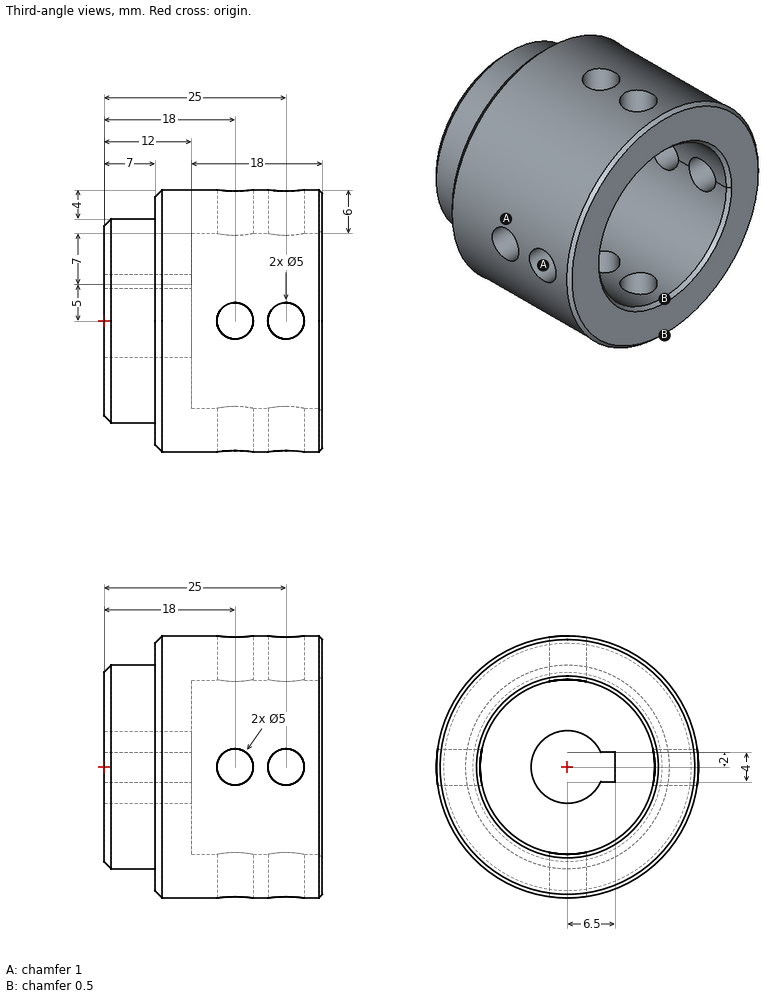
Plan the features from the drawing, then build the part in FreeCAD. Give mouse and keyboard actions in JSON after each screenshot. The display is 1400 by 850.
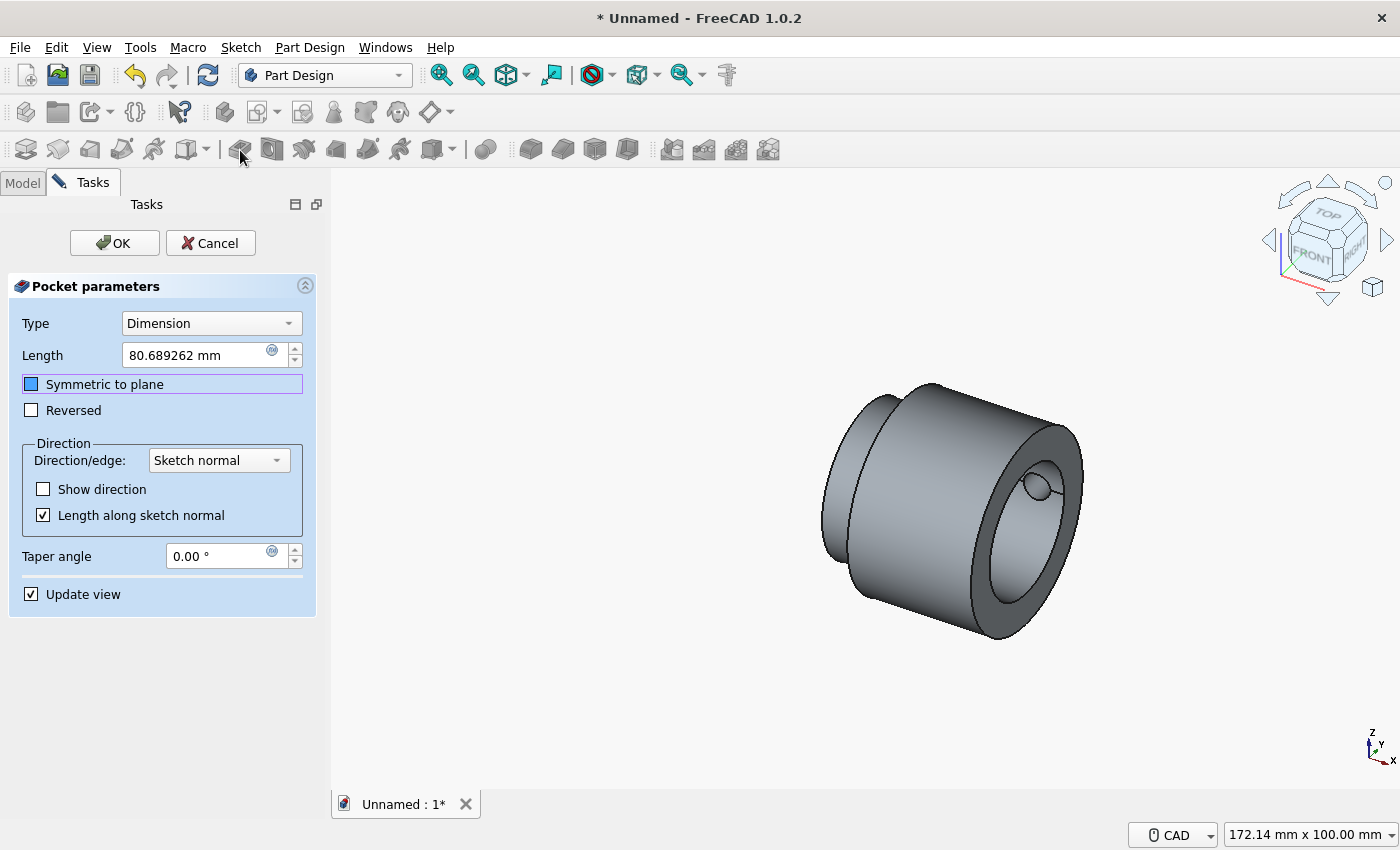
{"action": "left_click", "coordinate": [30, 384]}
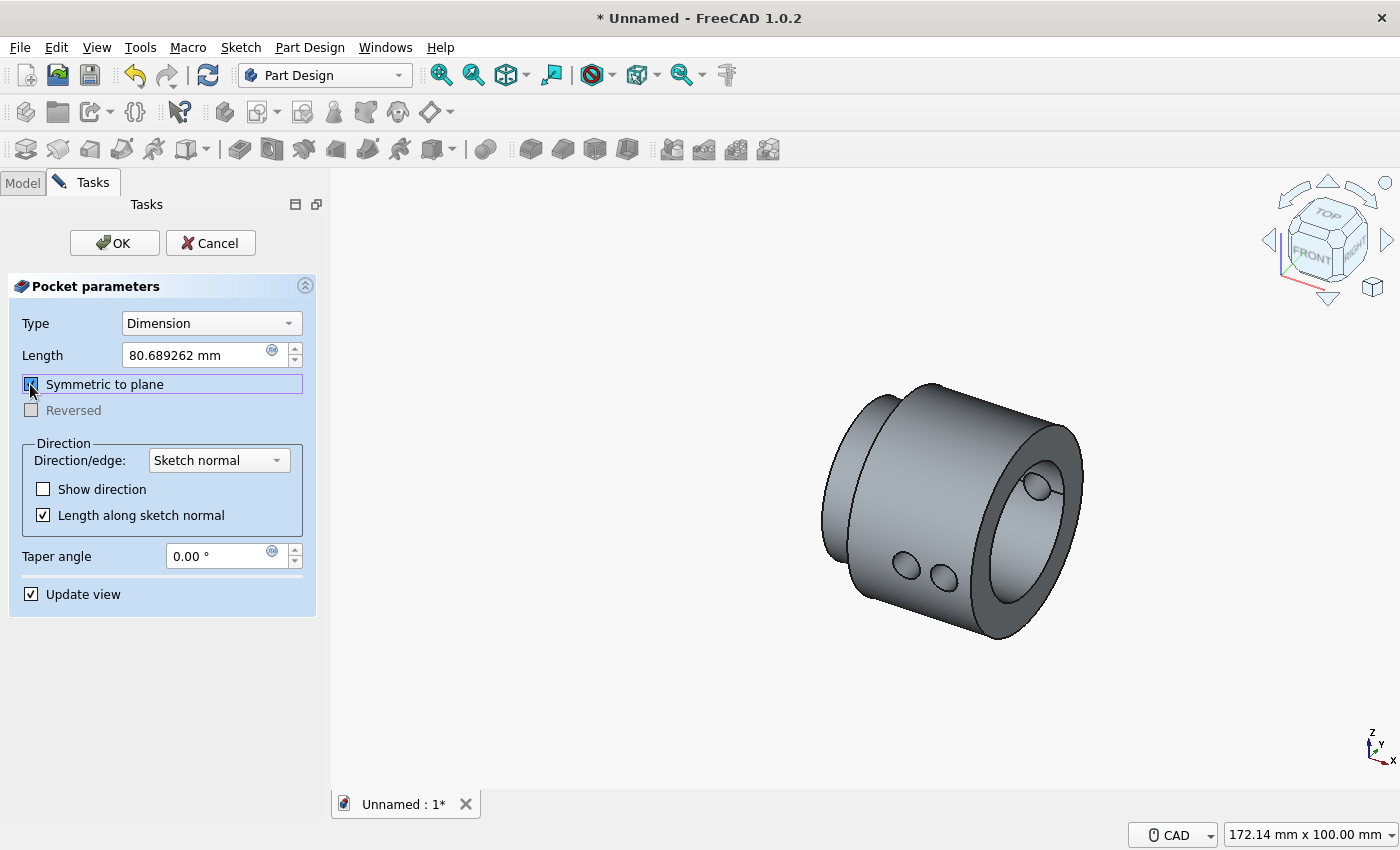
{"action": "left_click", "coordinate": [115, 243]}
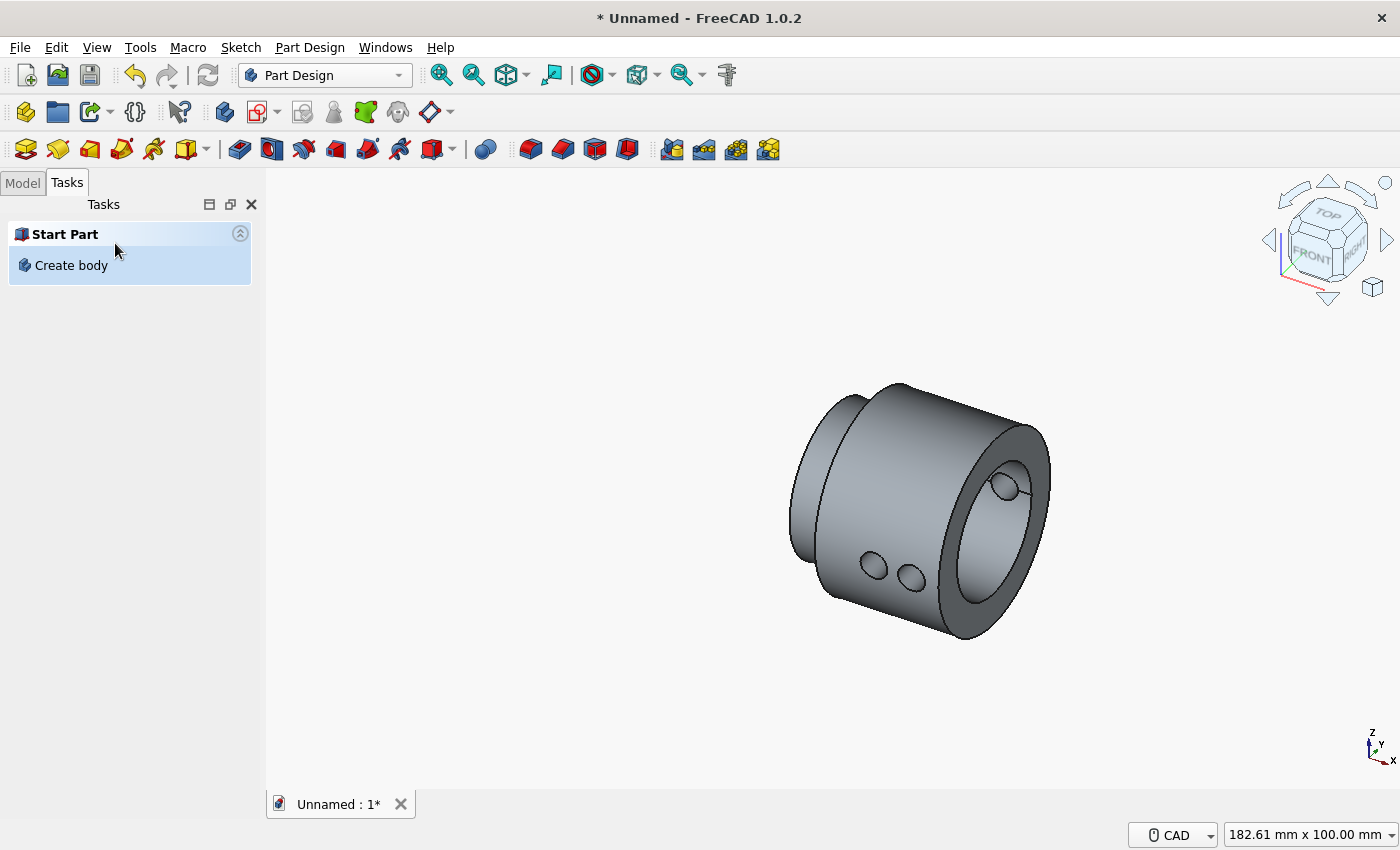
{"action": "left_click", "coordinate": [820, 423]}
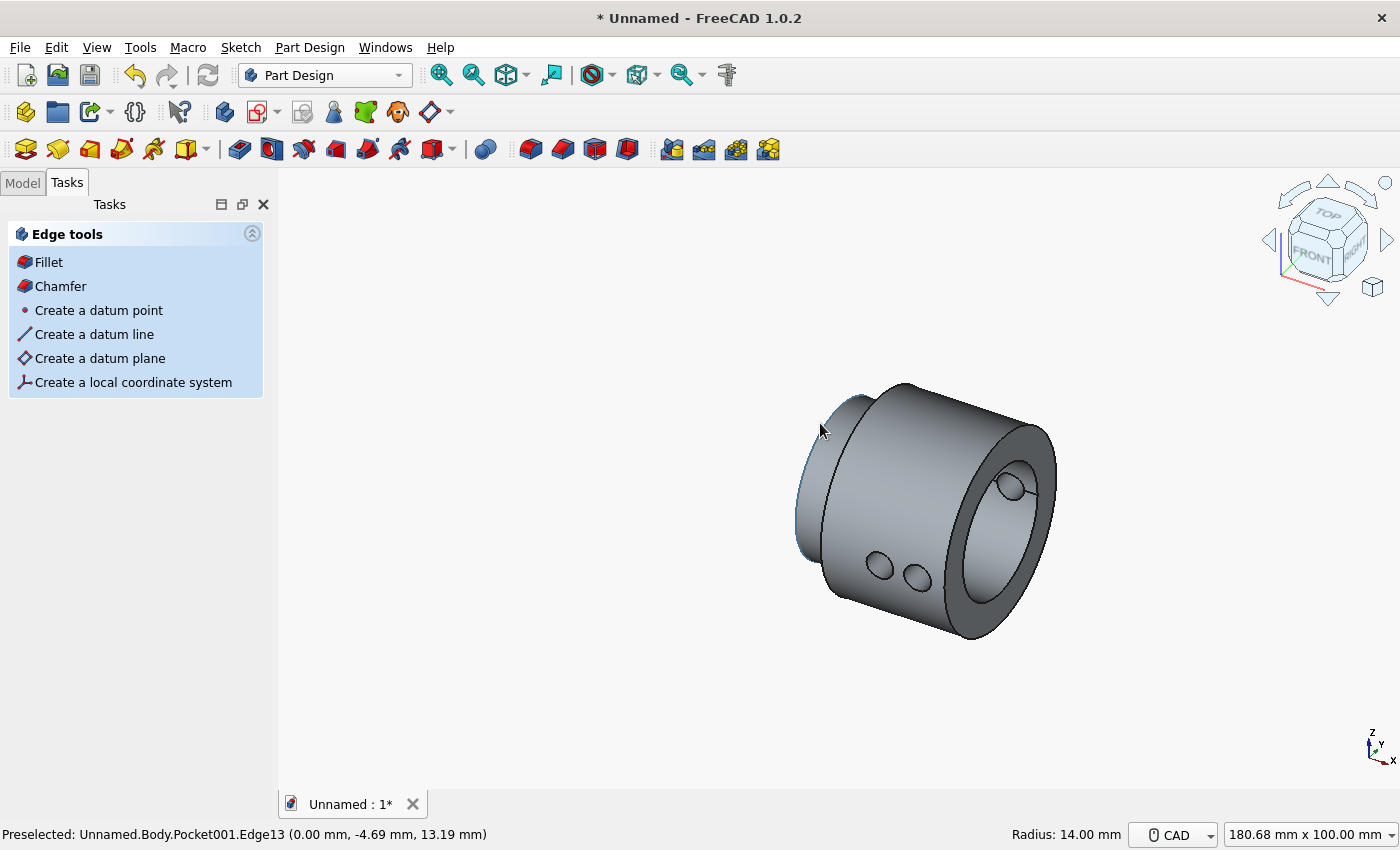
{"action": "left_click", "coordinate": [859, 420], "text": "ctrl"}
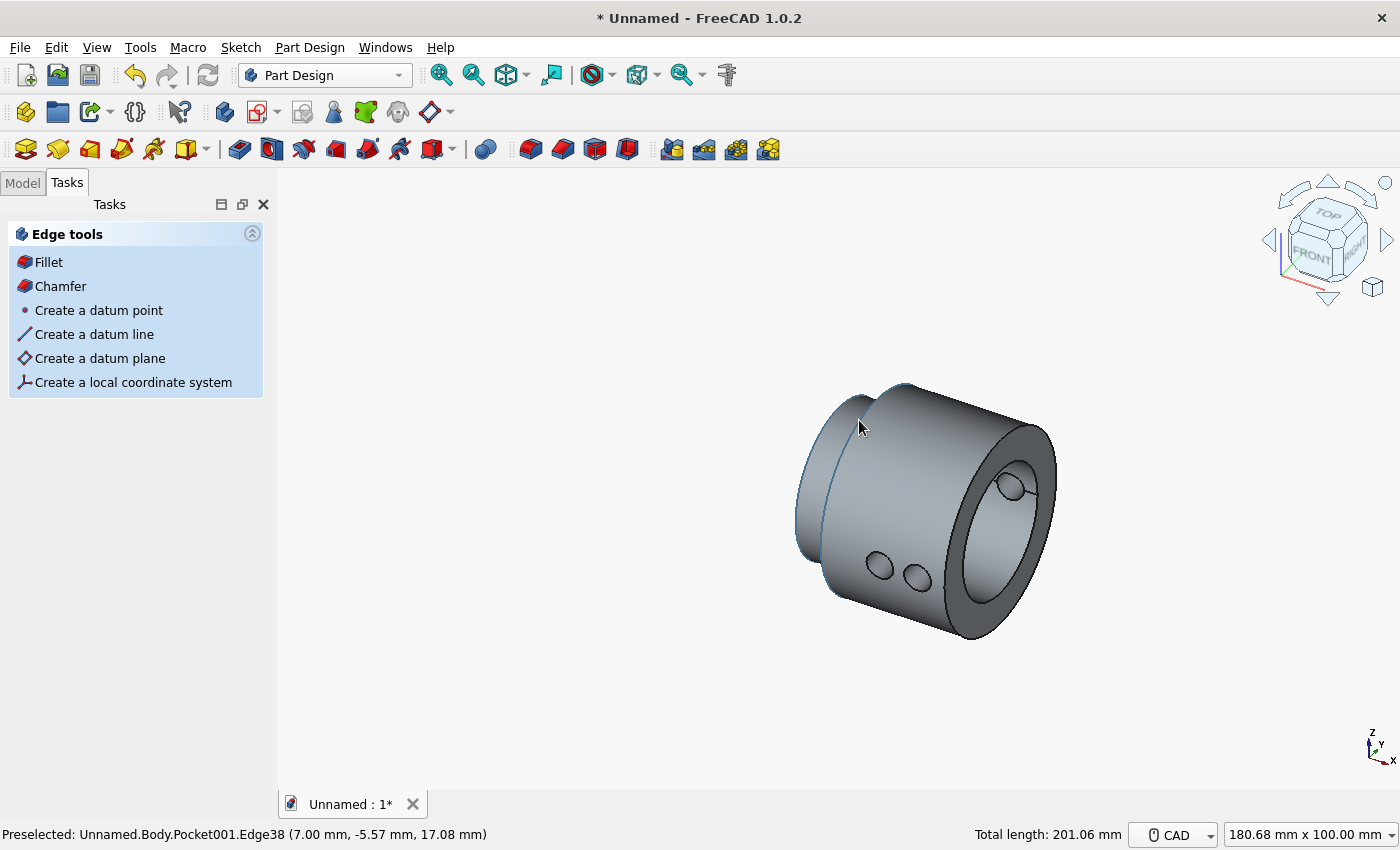
{"action": "left_click", "coordinate": [564, 150]}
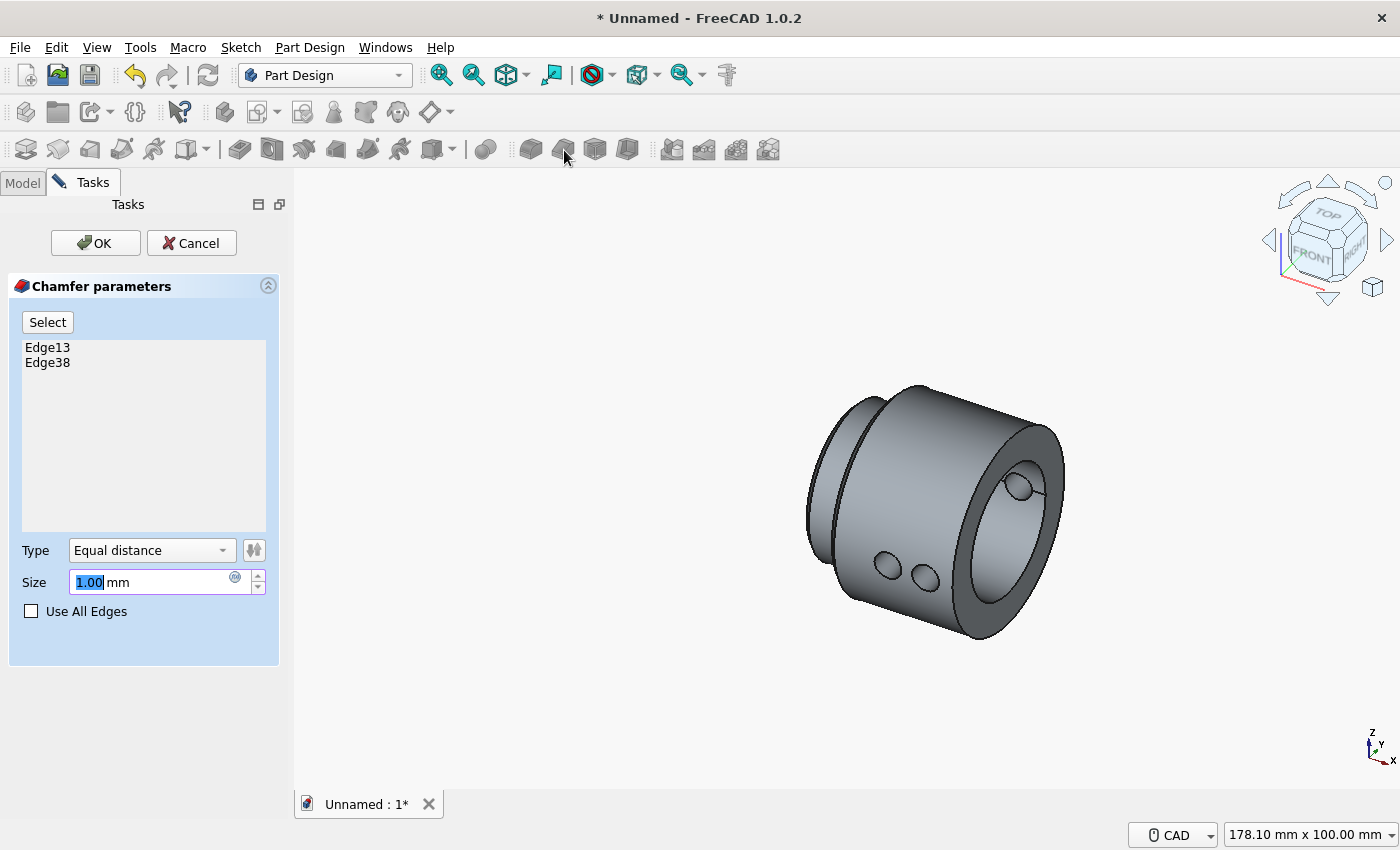
{"action": "type", "text": "1"}
{"action": "key", "text": "Tab"}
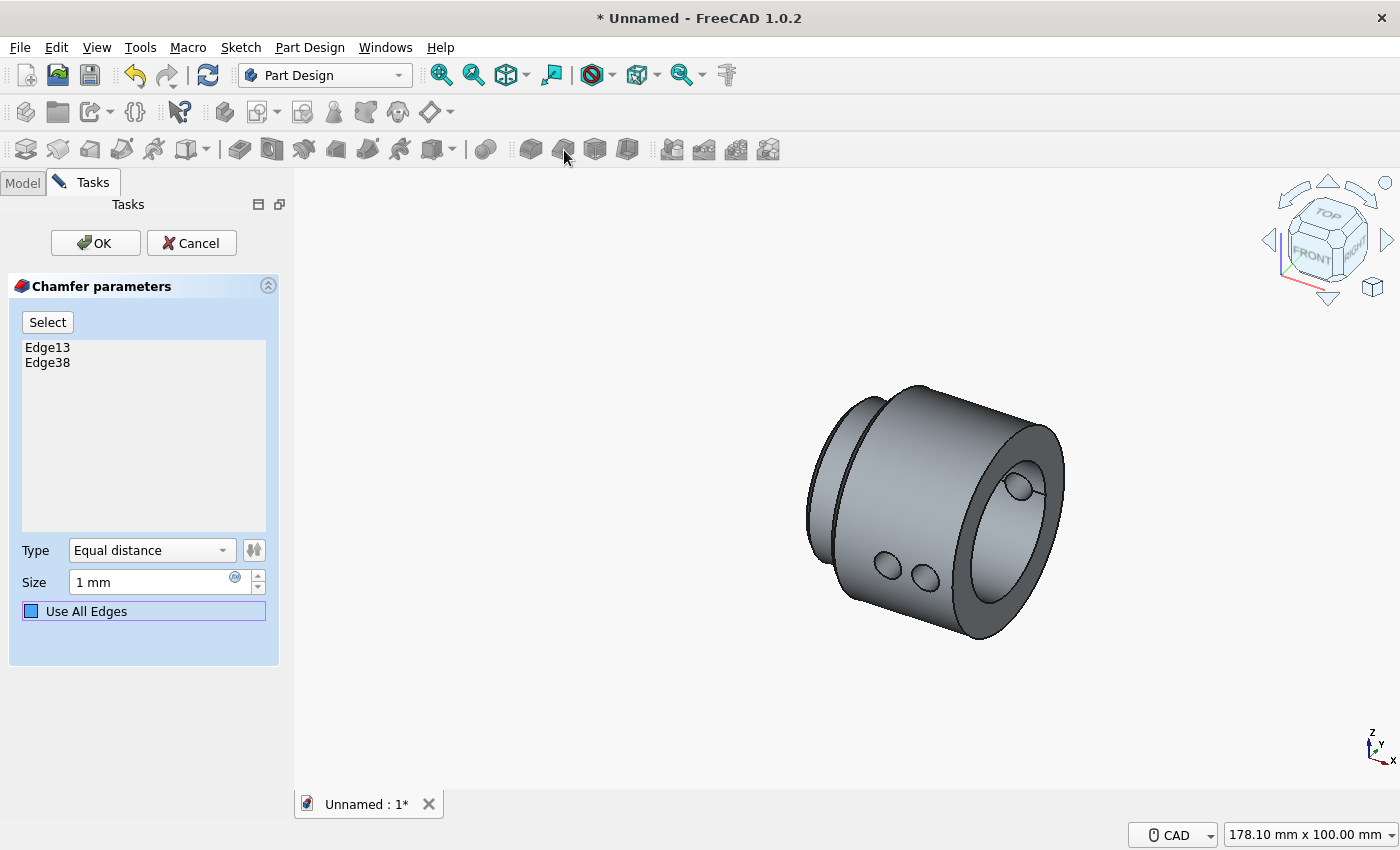
{"action": "left_click", "coordinate": [96, 243]}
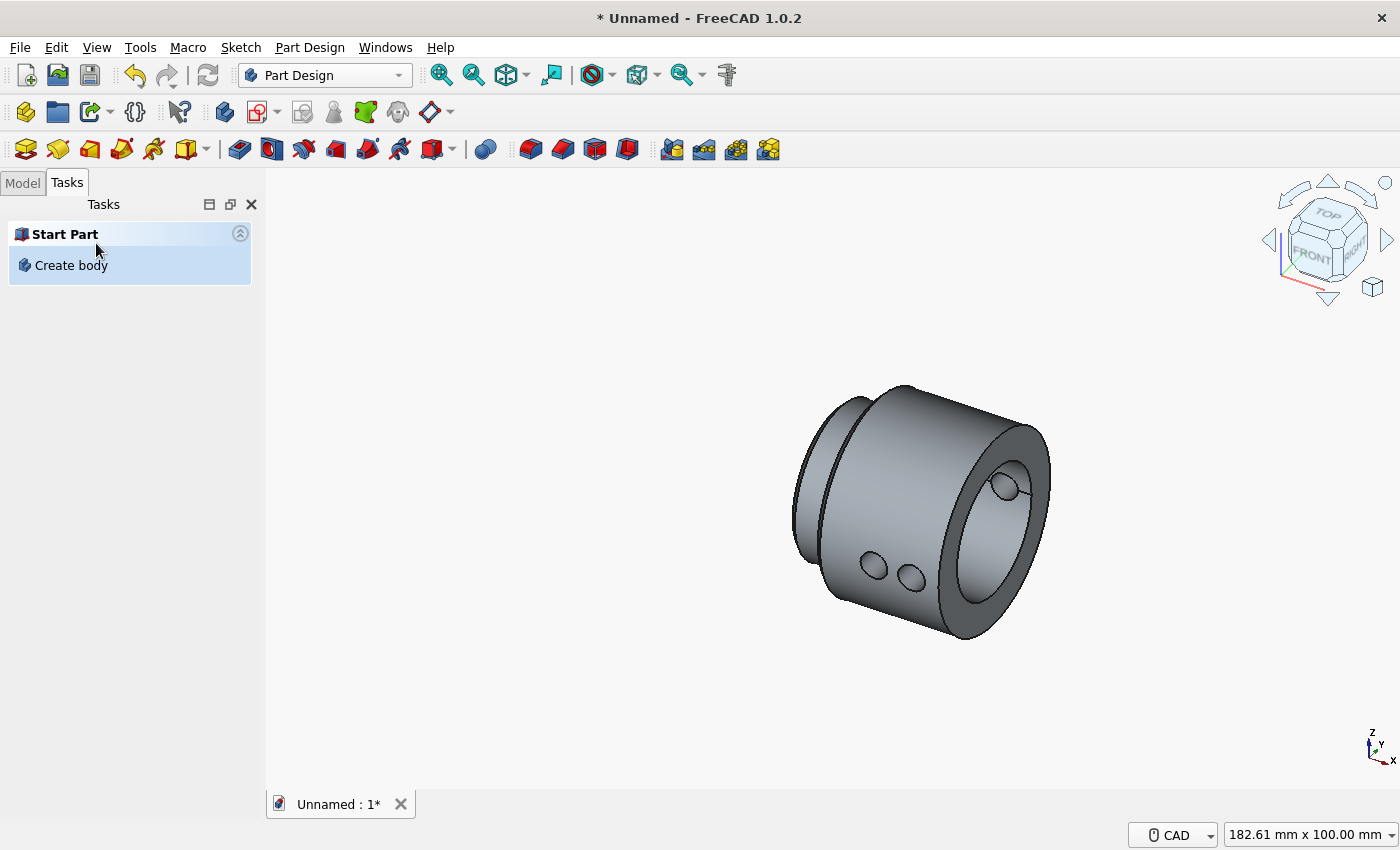
{"action": "left_click", "coordinate": [938, 586]}